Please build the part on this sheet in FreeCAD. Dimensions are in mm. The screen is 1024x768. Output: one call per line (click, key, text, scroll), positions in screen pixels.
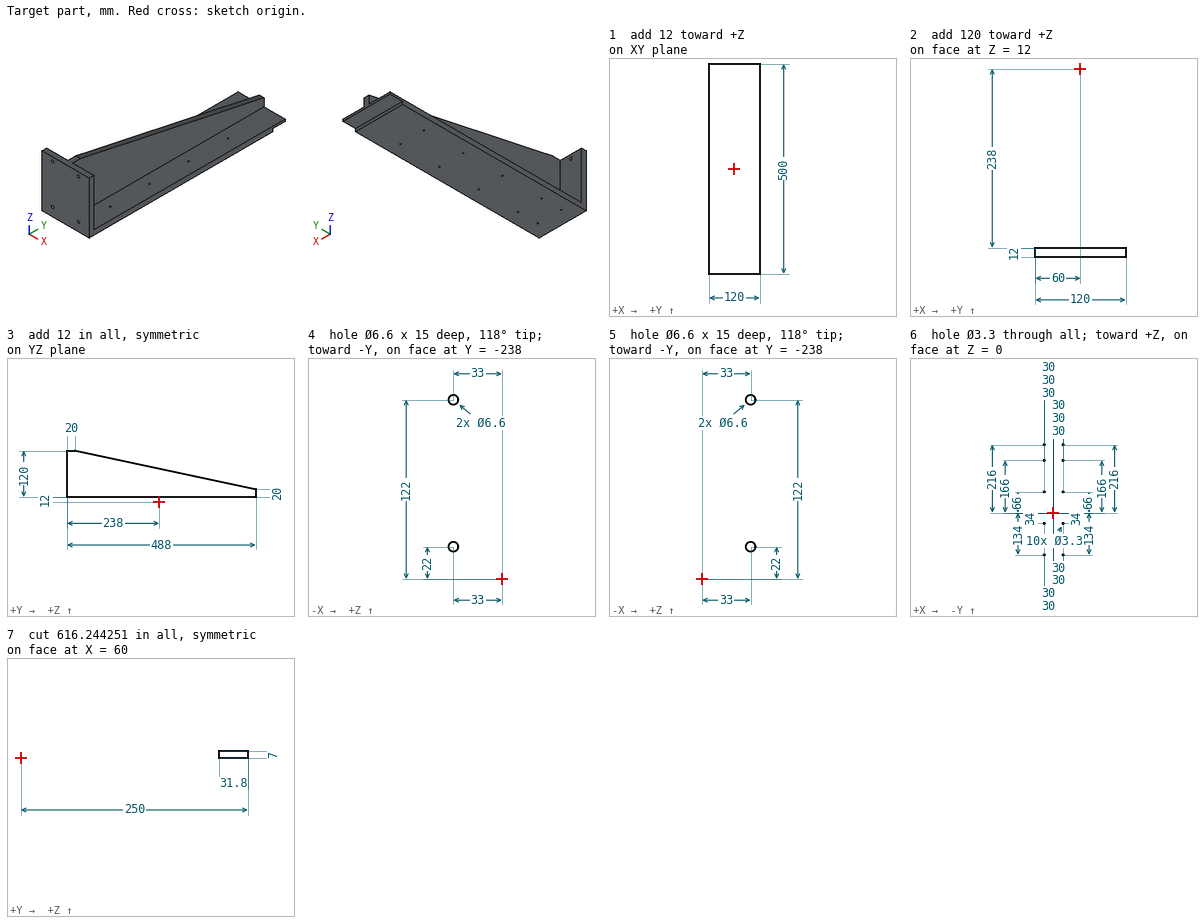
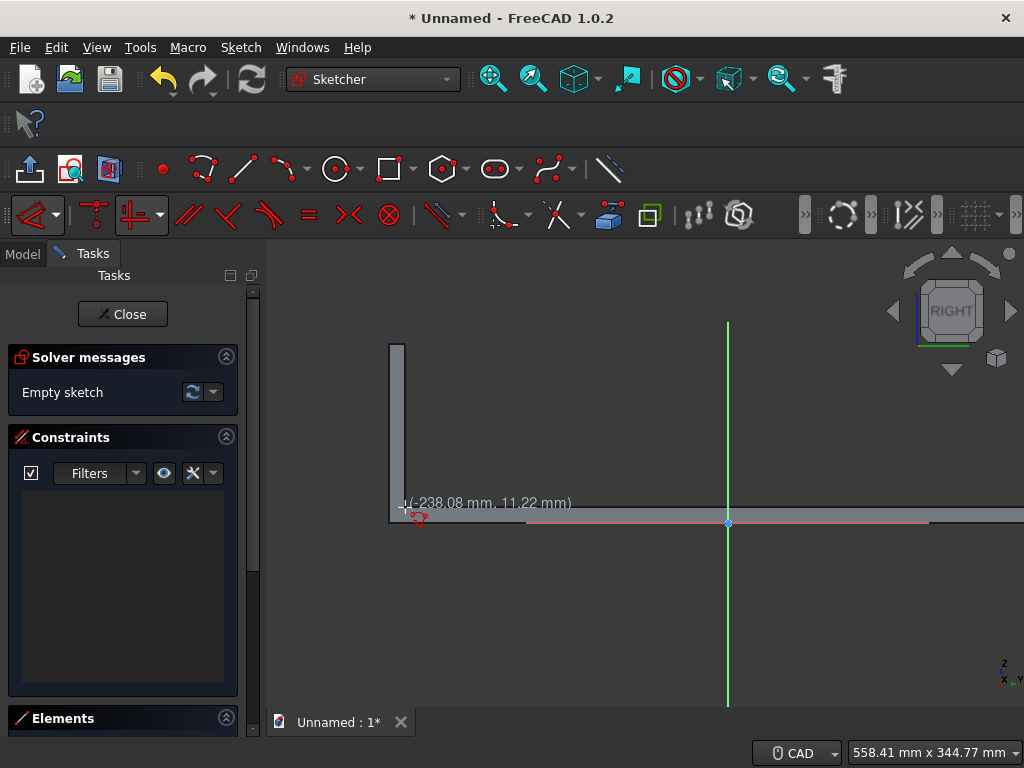
scroll(382, 521, down, 3)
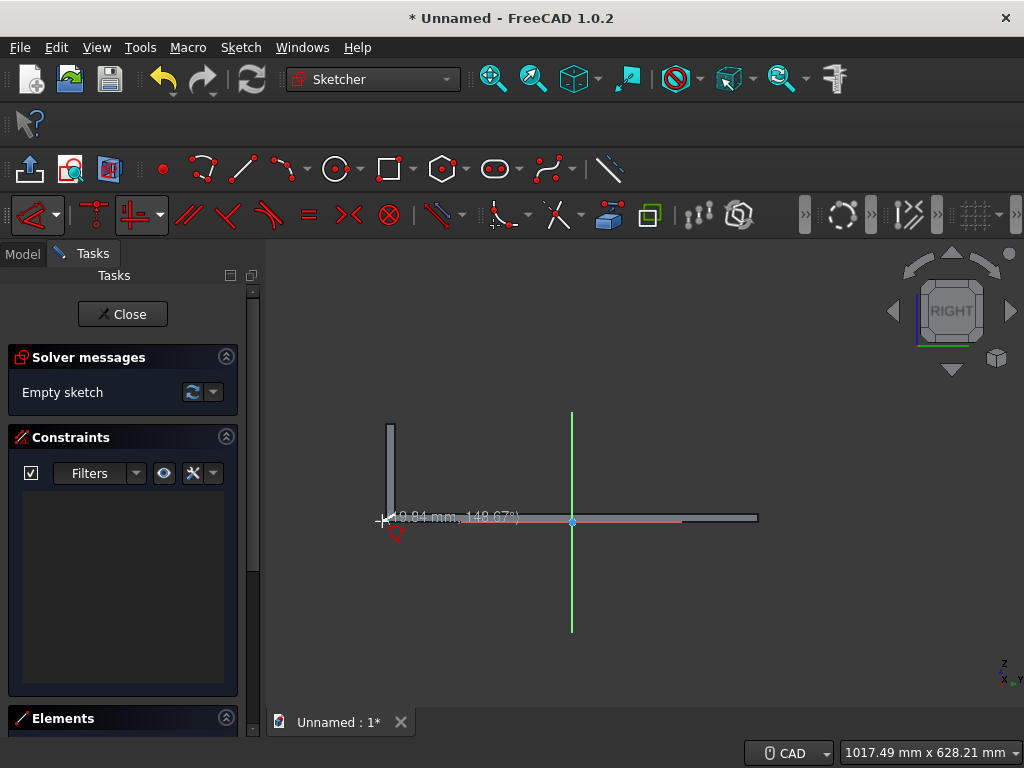
scroll(758, 514, up, 3)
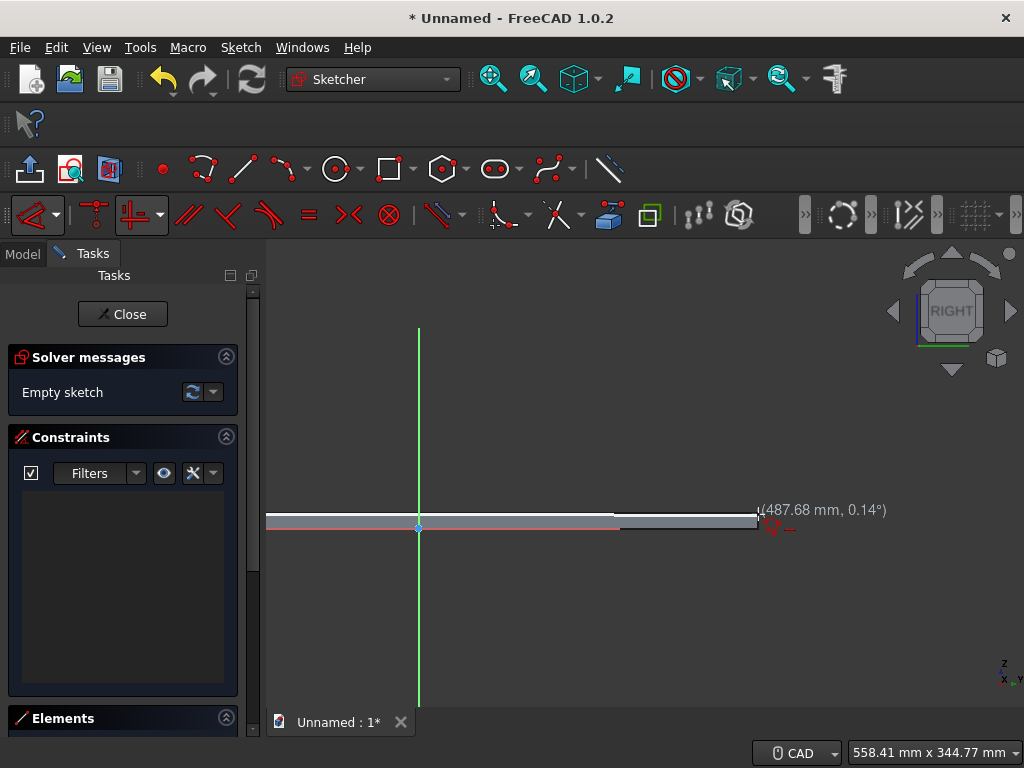
click(758, 513)
click(758, 486)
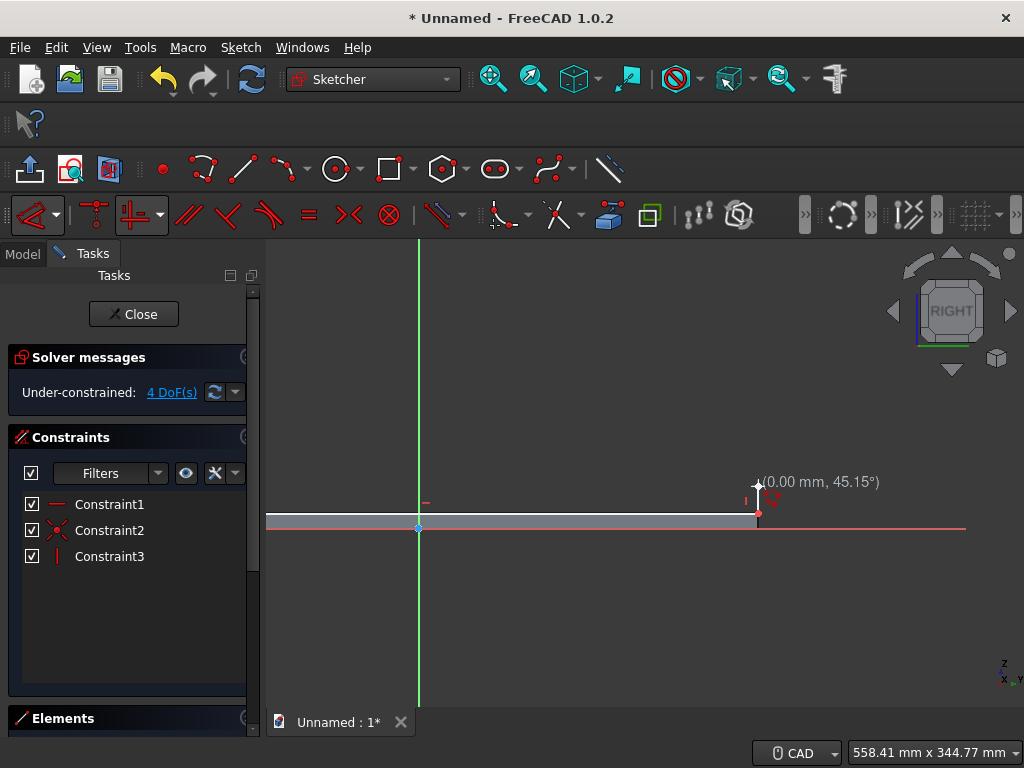
scroll(759, 514, down, 3)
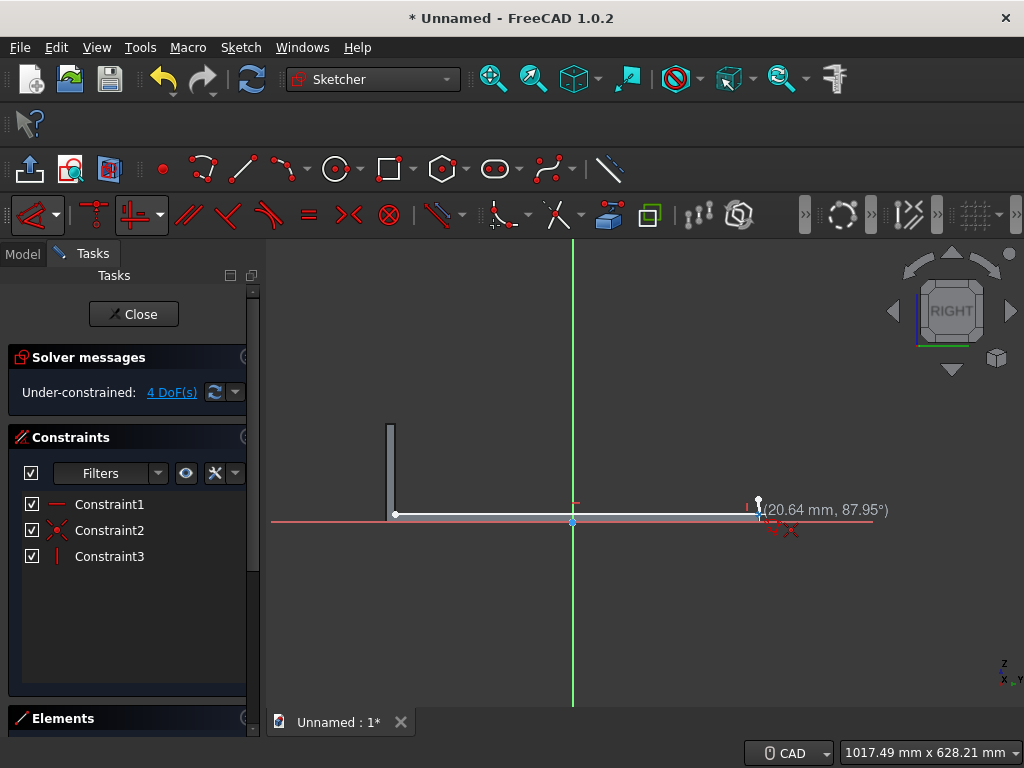
click(410, 424)
click(395, 424)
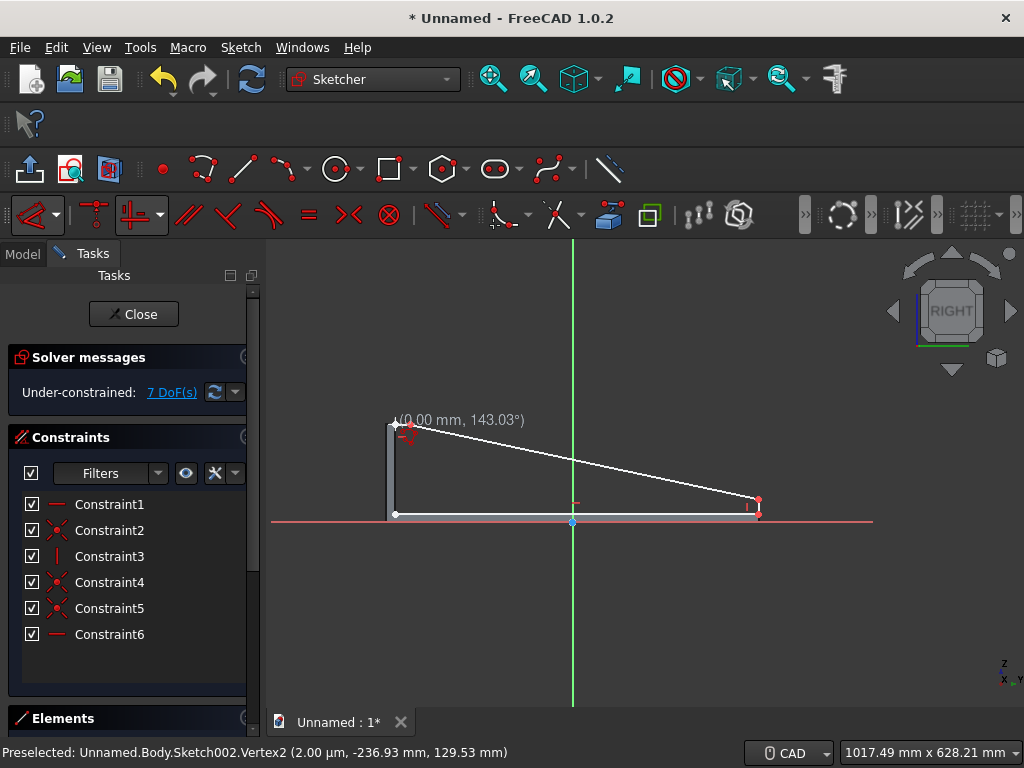
scroll(395, 514, up, 3)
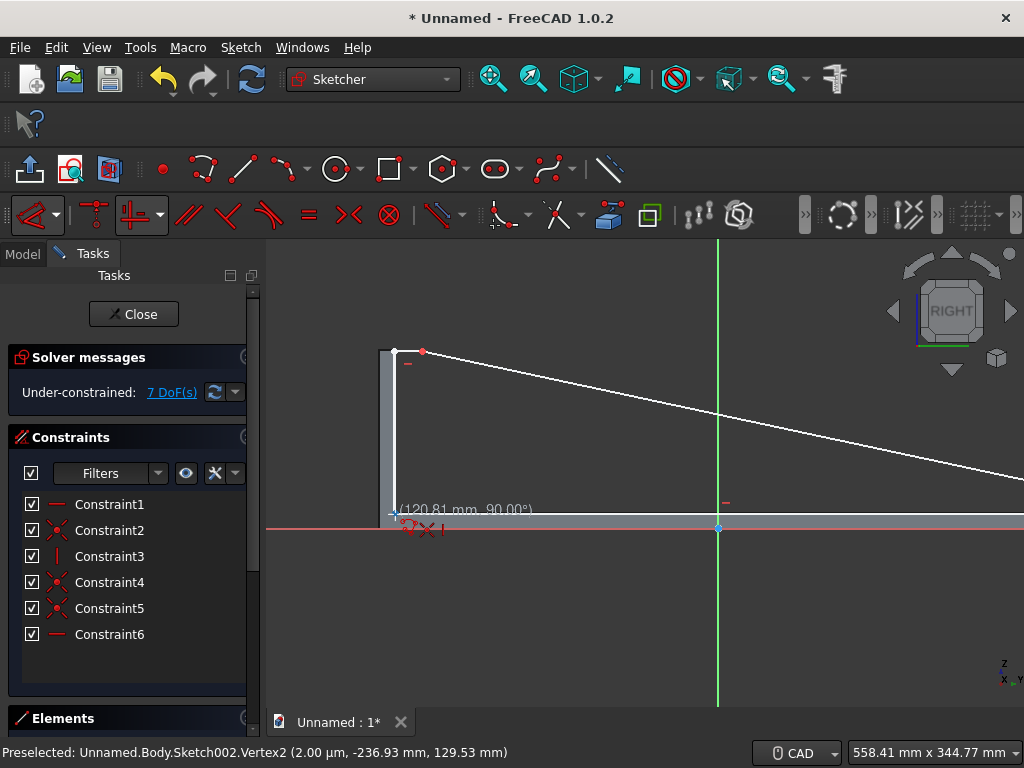
click(395, 514)
key(Escape)
key(Escape)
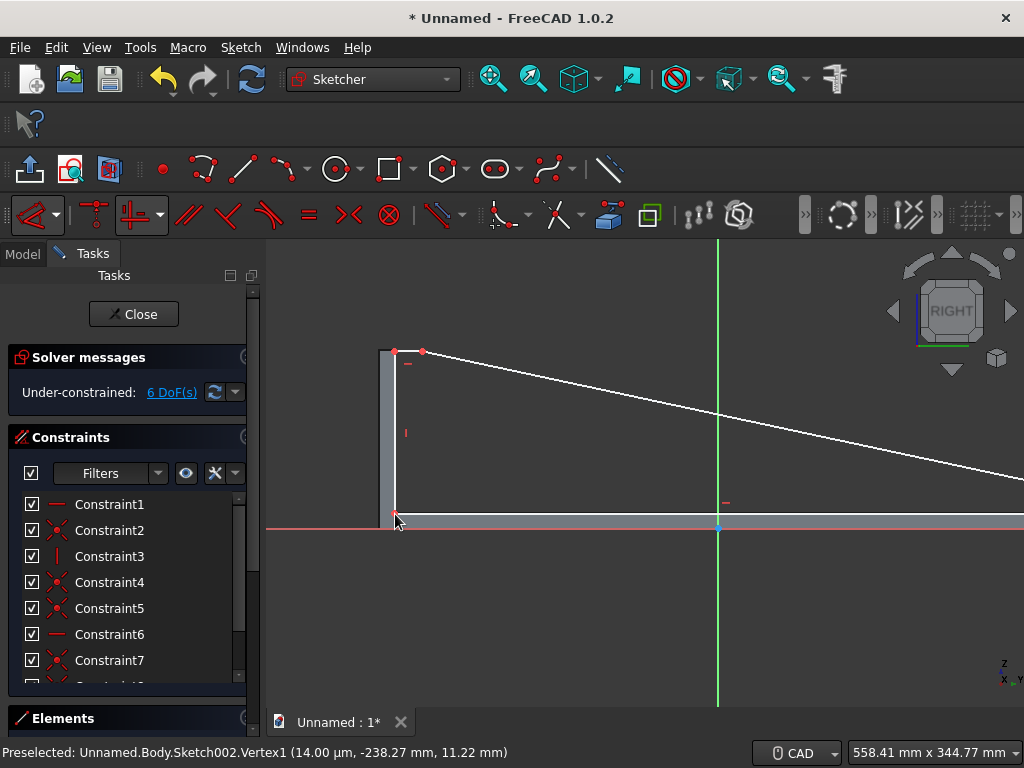
scroll(394, 514, down, 3)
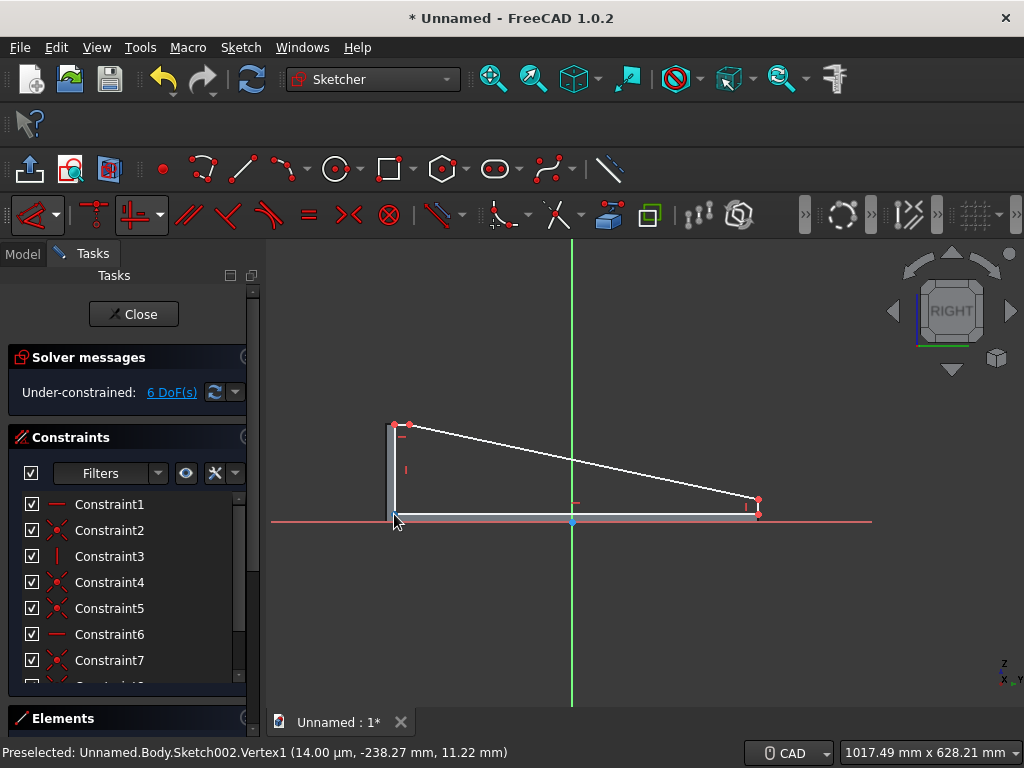
scroll(758, 508, up, 5)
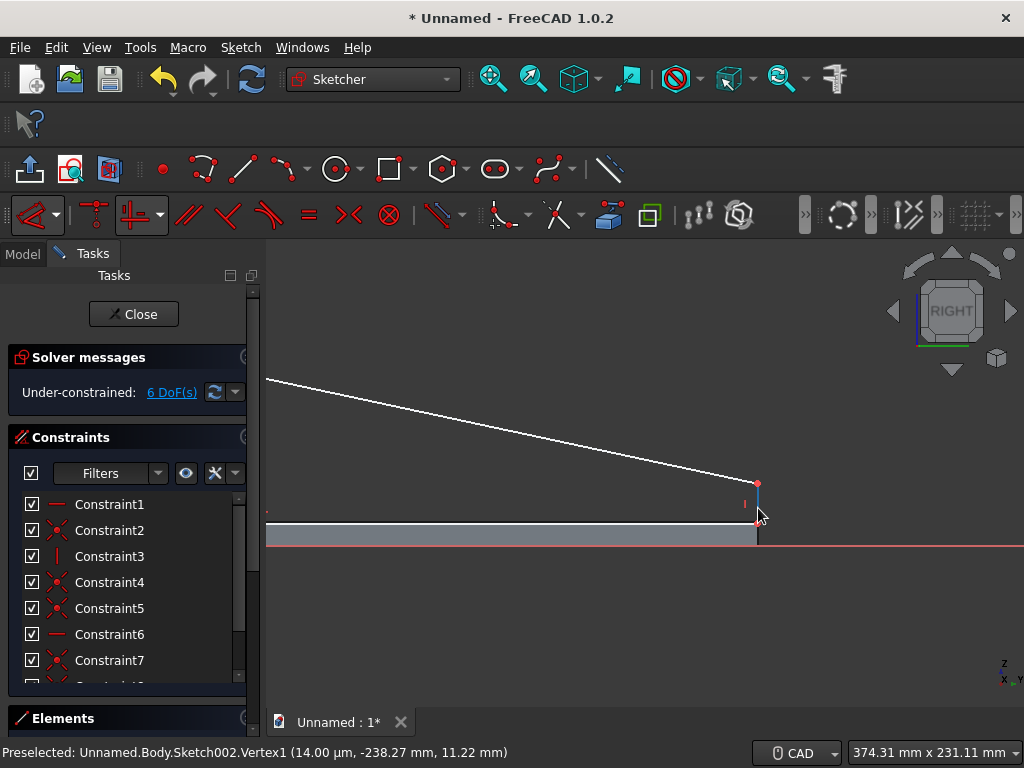
click(758, 508)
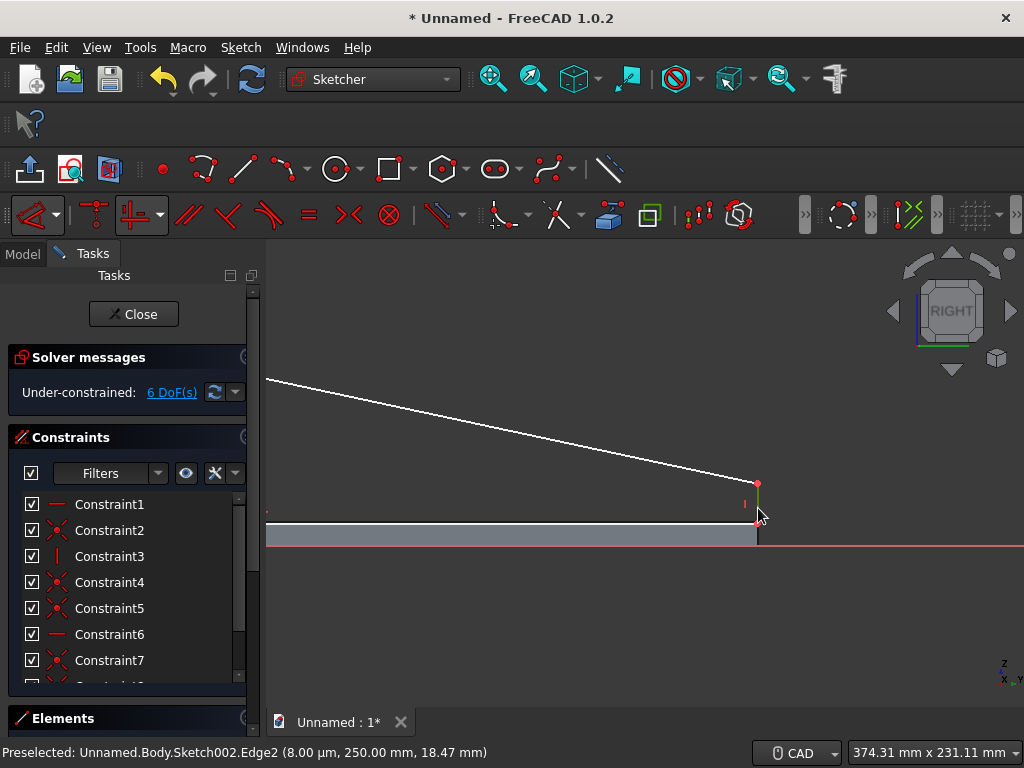
click(58, 216)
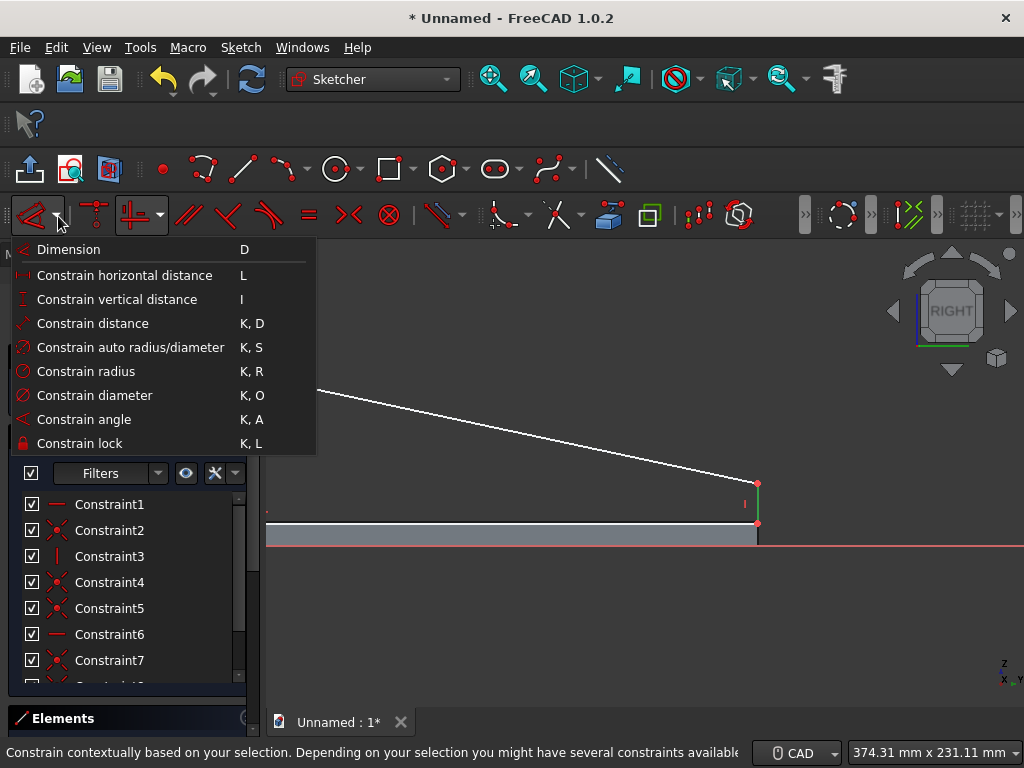
click(164, 299)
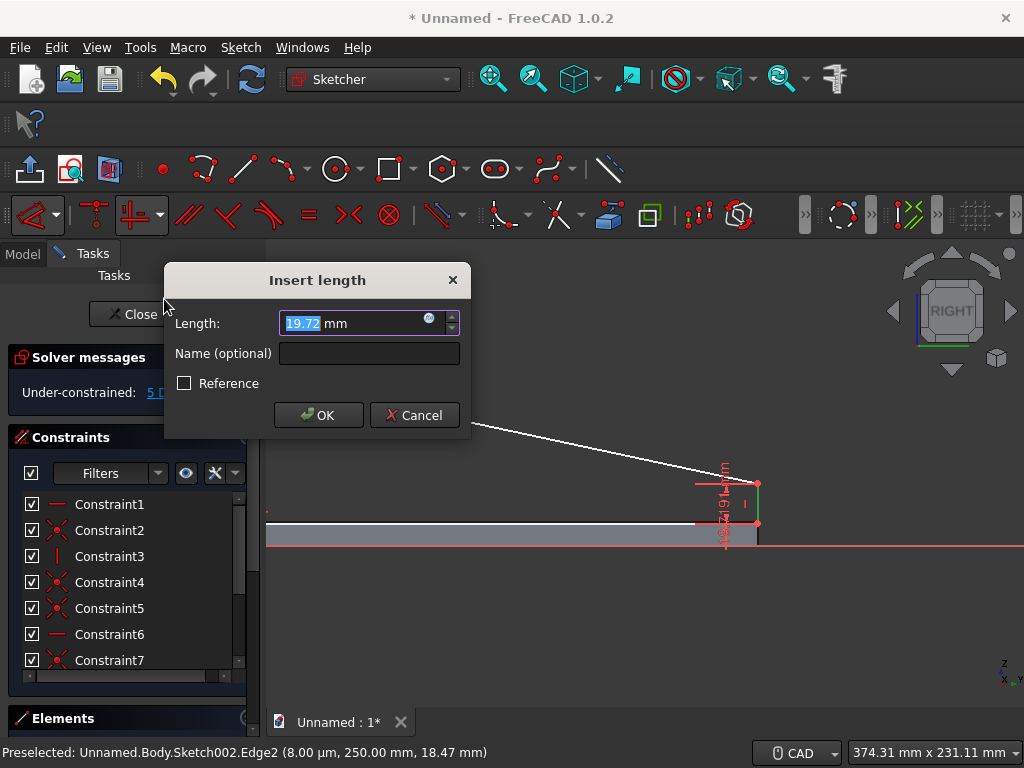
text(20)
key(Return)